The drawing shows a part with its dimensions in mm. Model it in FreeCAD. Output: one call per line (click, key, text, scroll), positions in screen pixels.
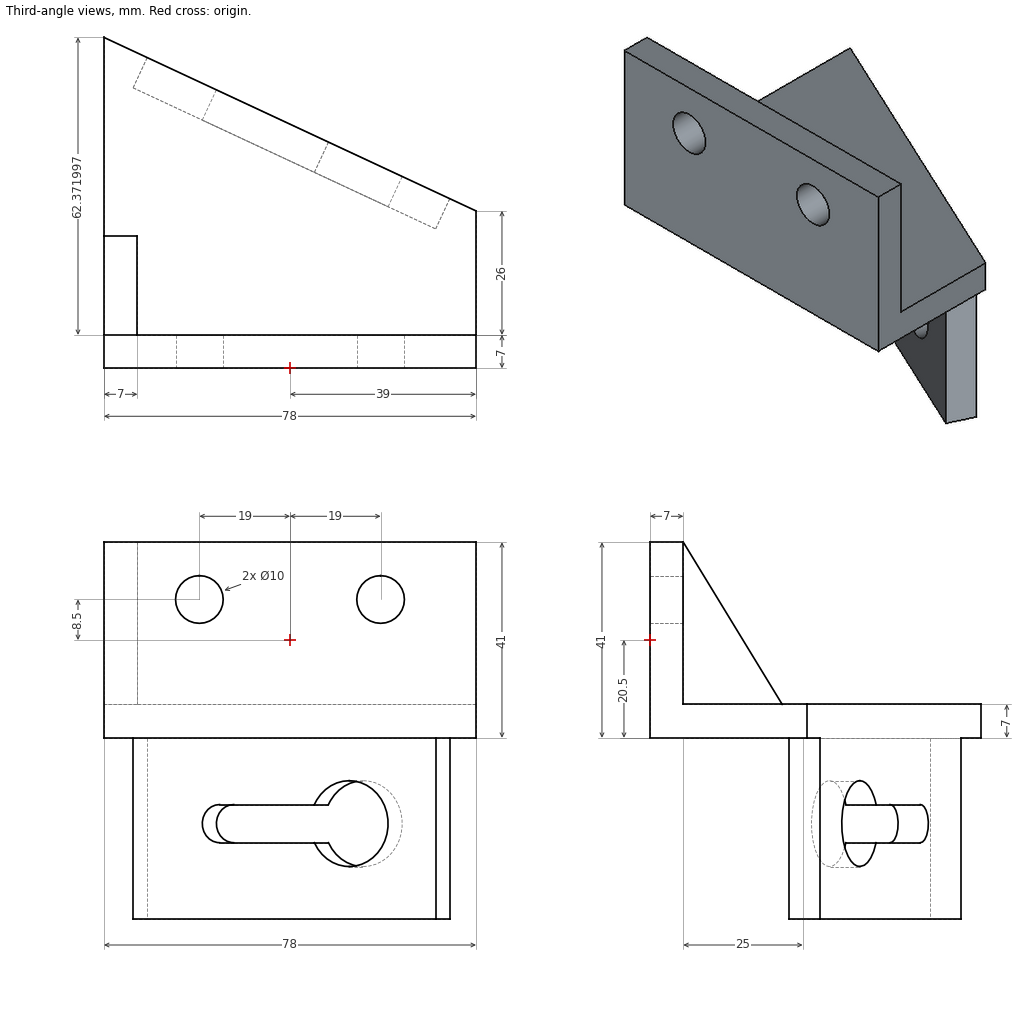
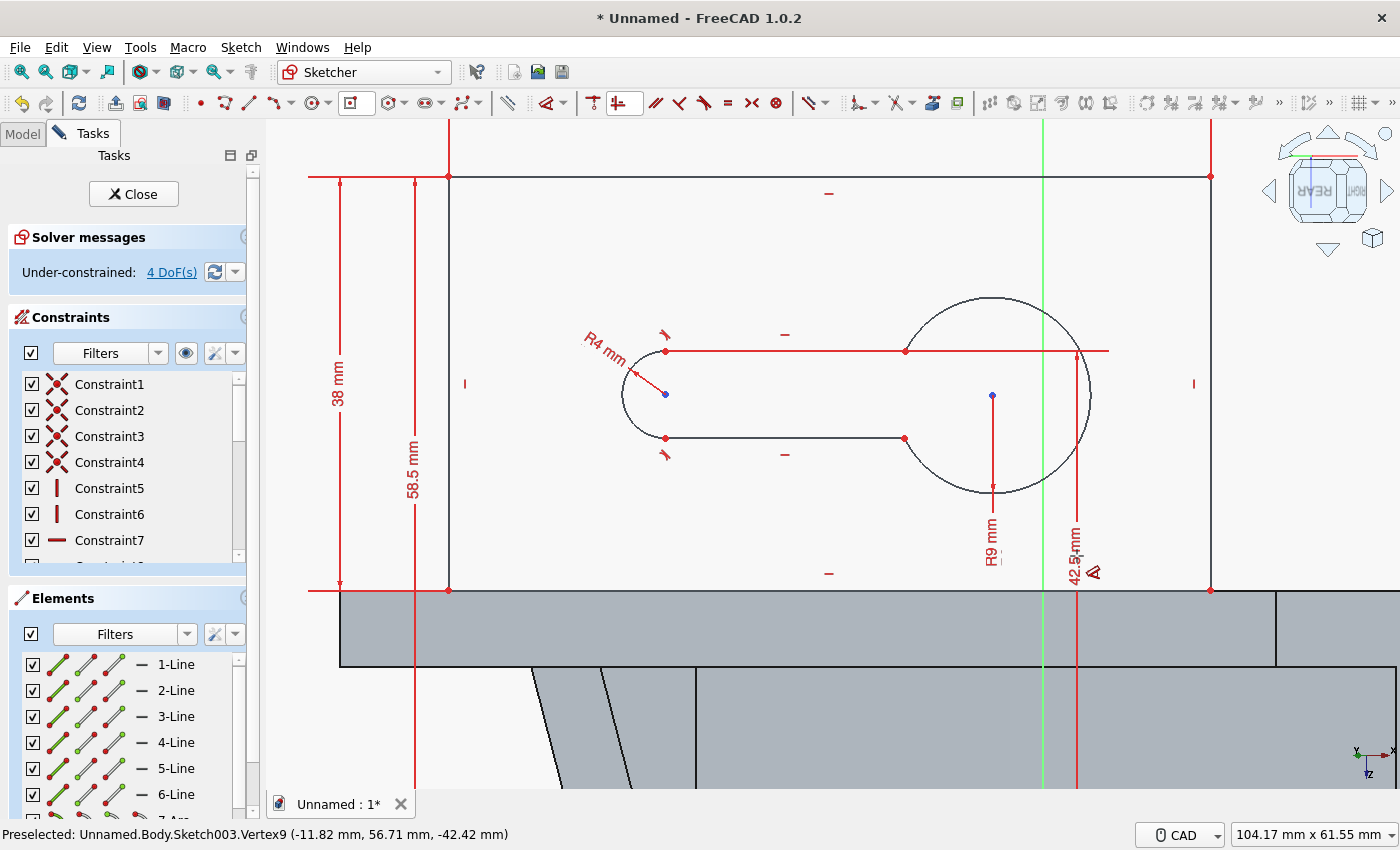
click(993, 396)
click(1077, 494)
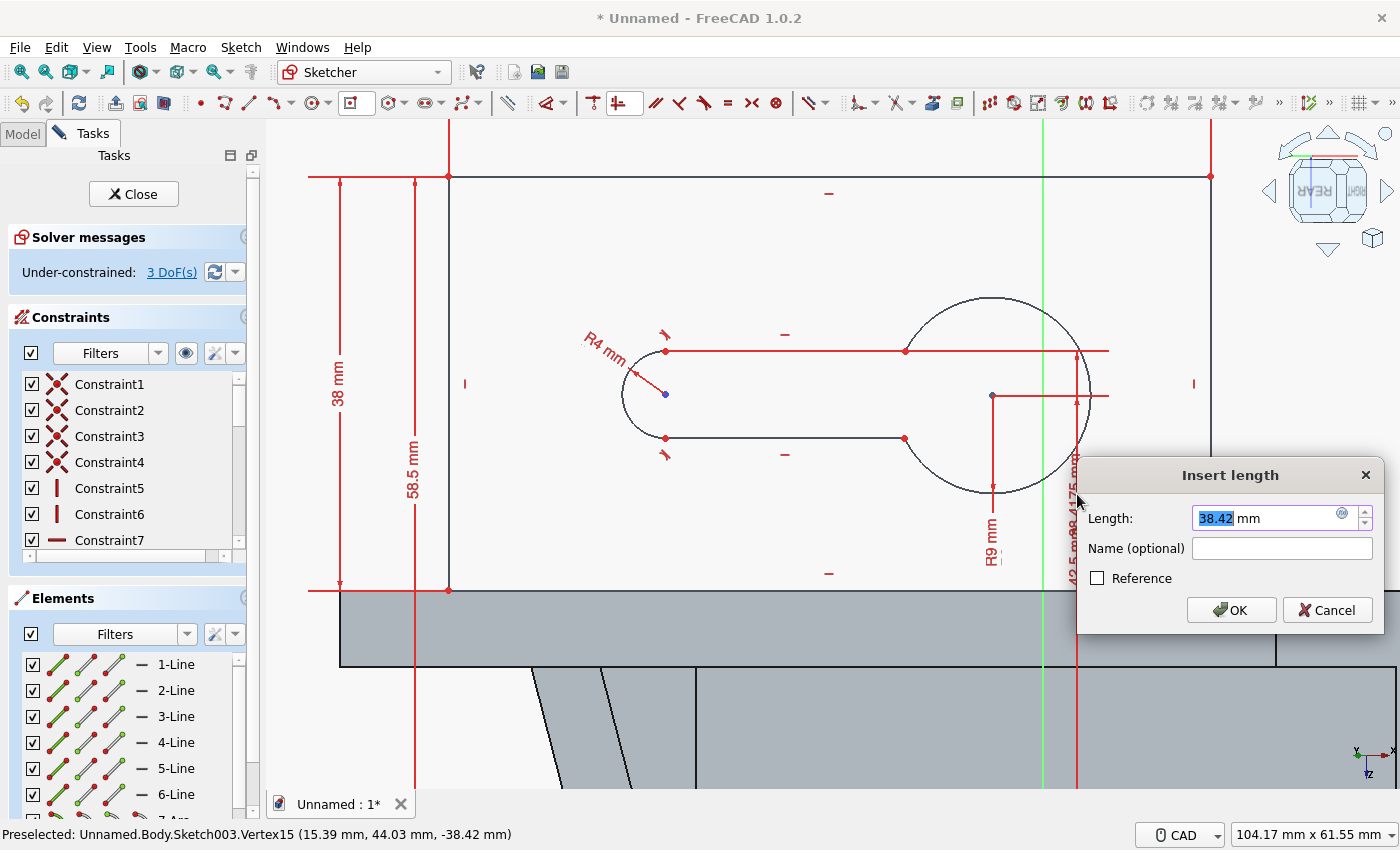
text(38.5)
key(Return)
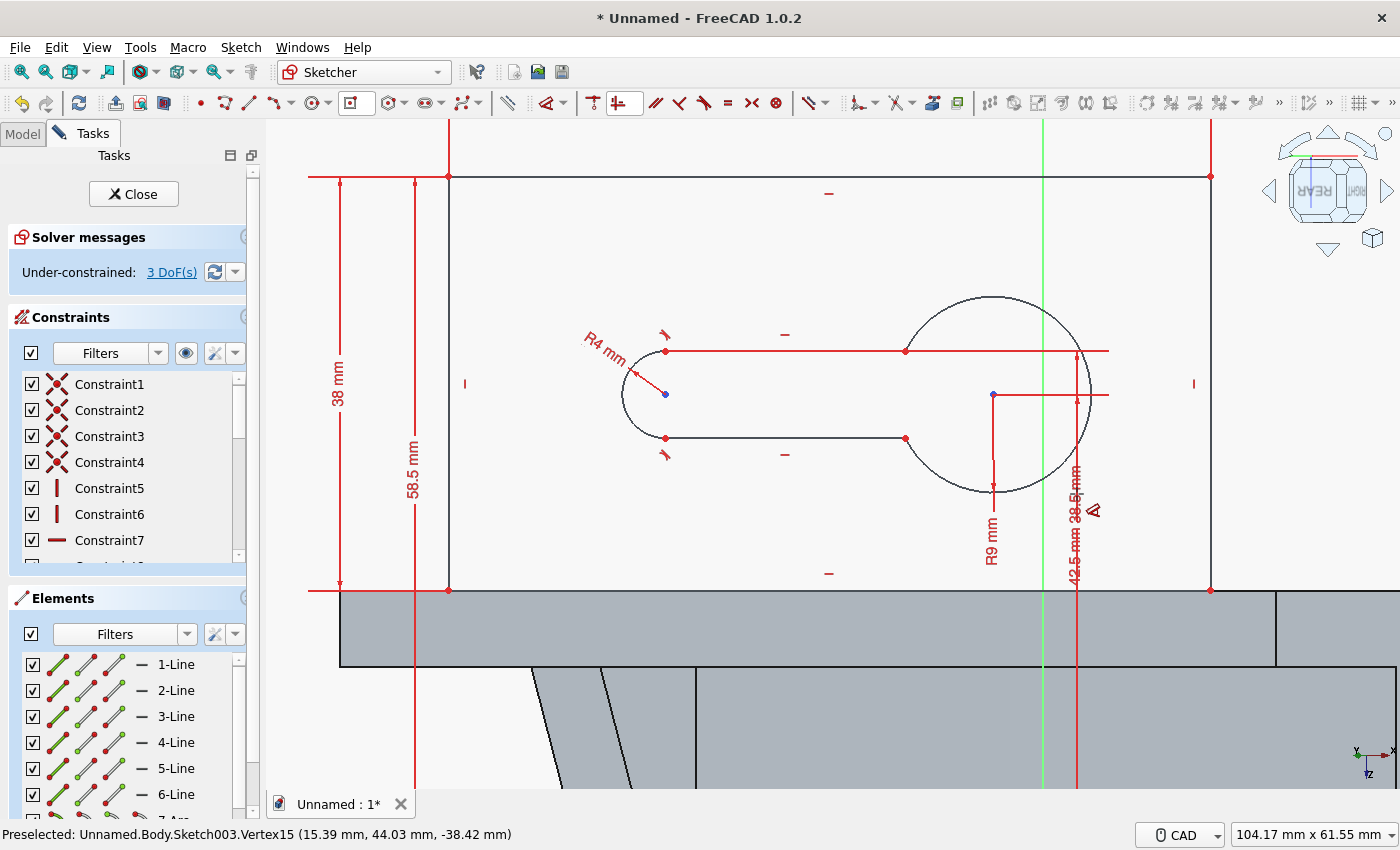
click(738, 351)
click(786, 317)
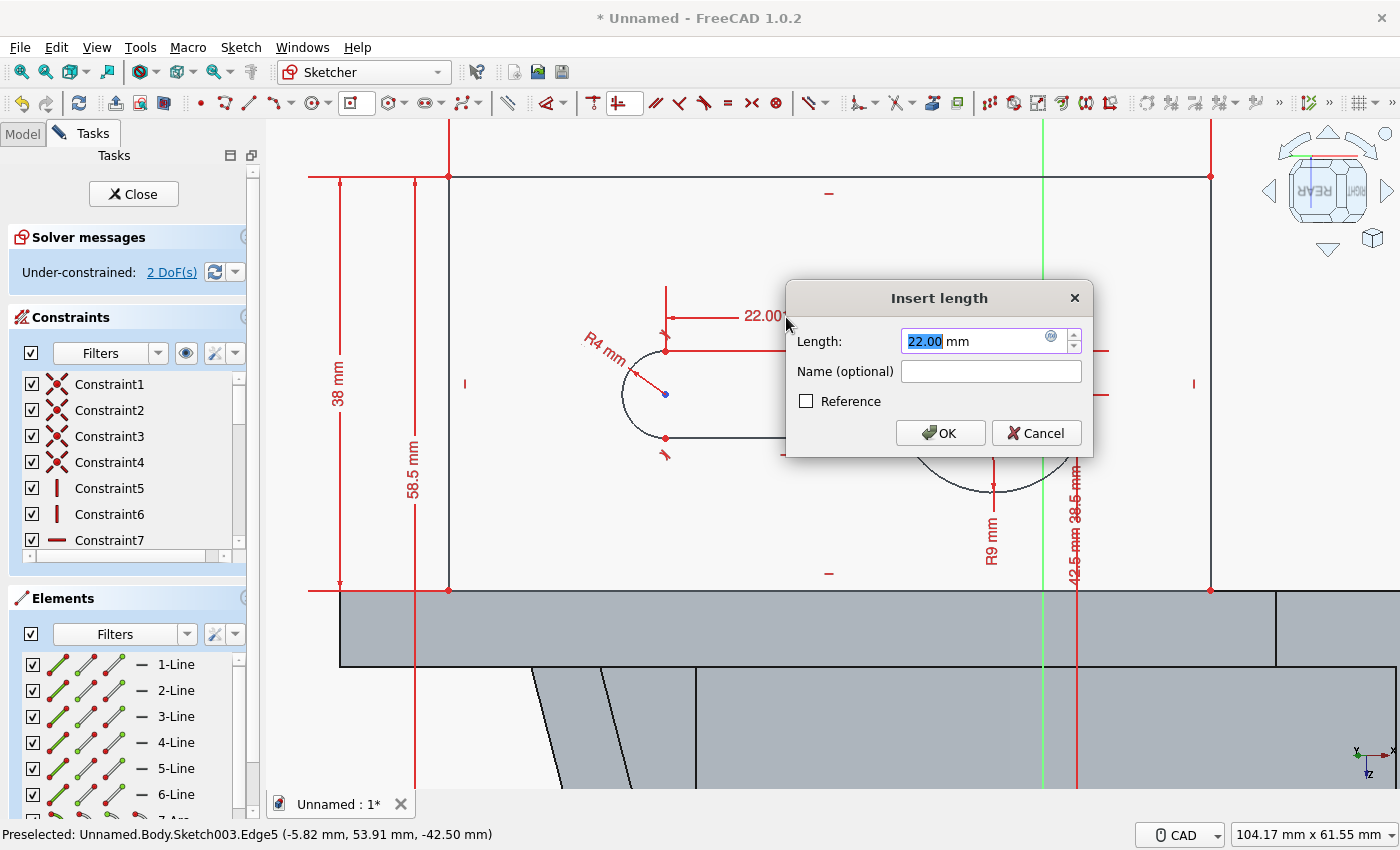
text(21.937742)
key(Return)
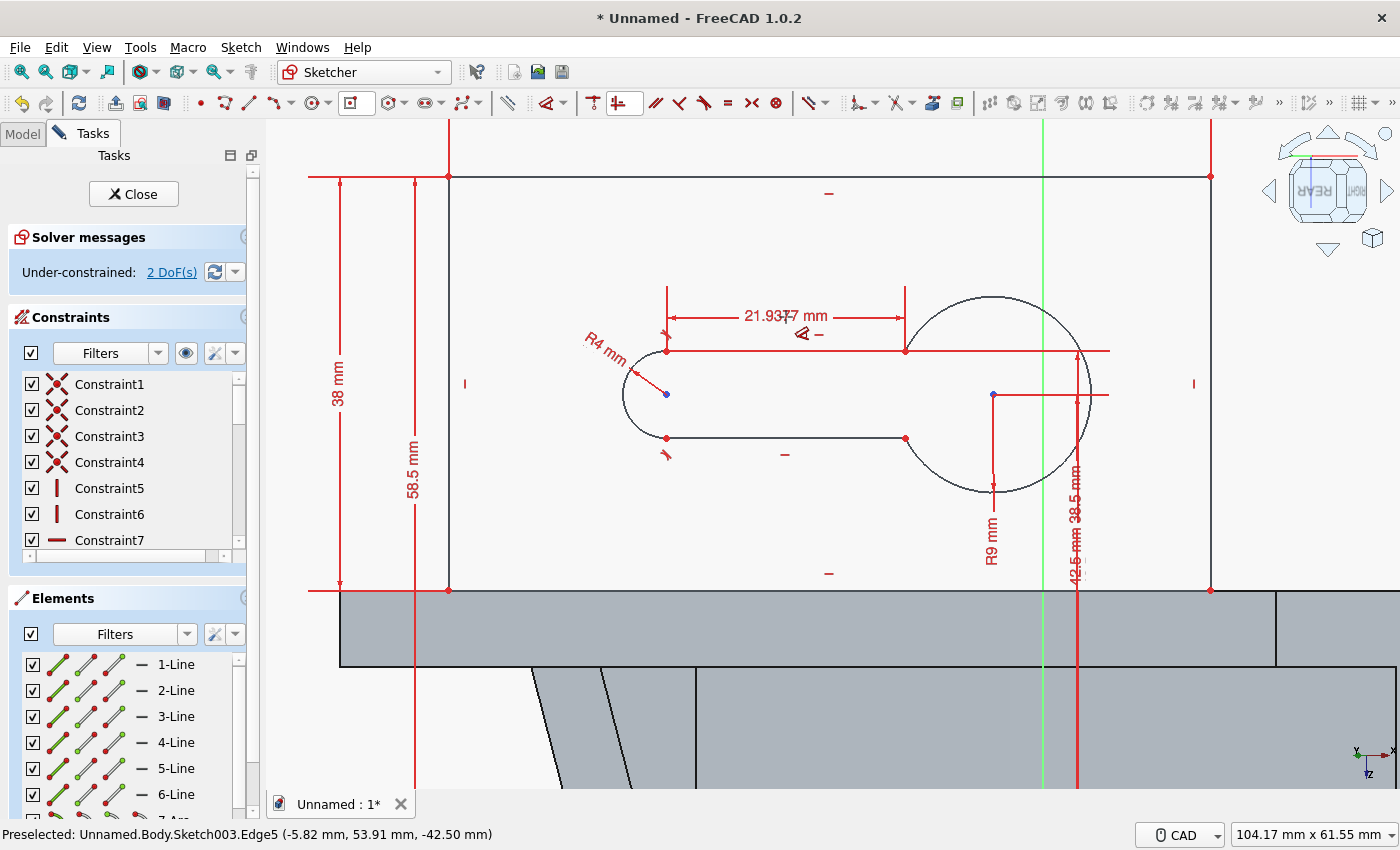
click(993, 395)
click(1018, 361)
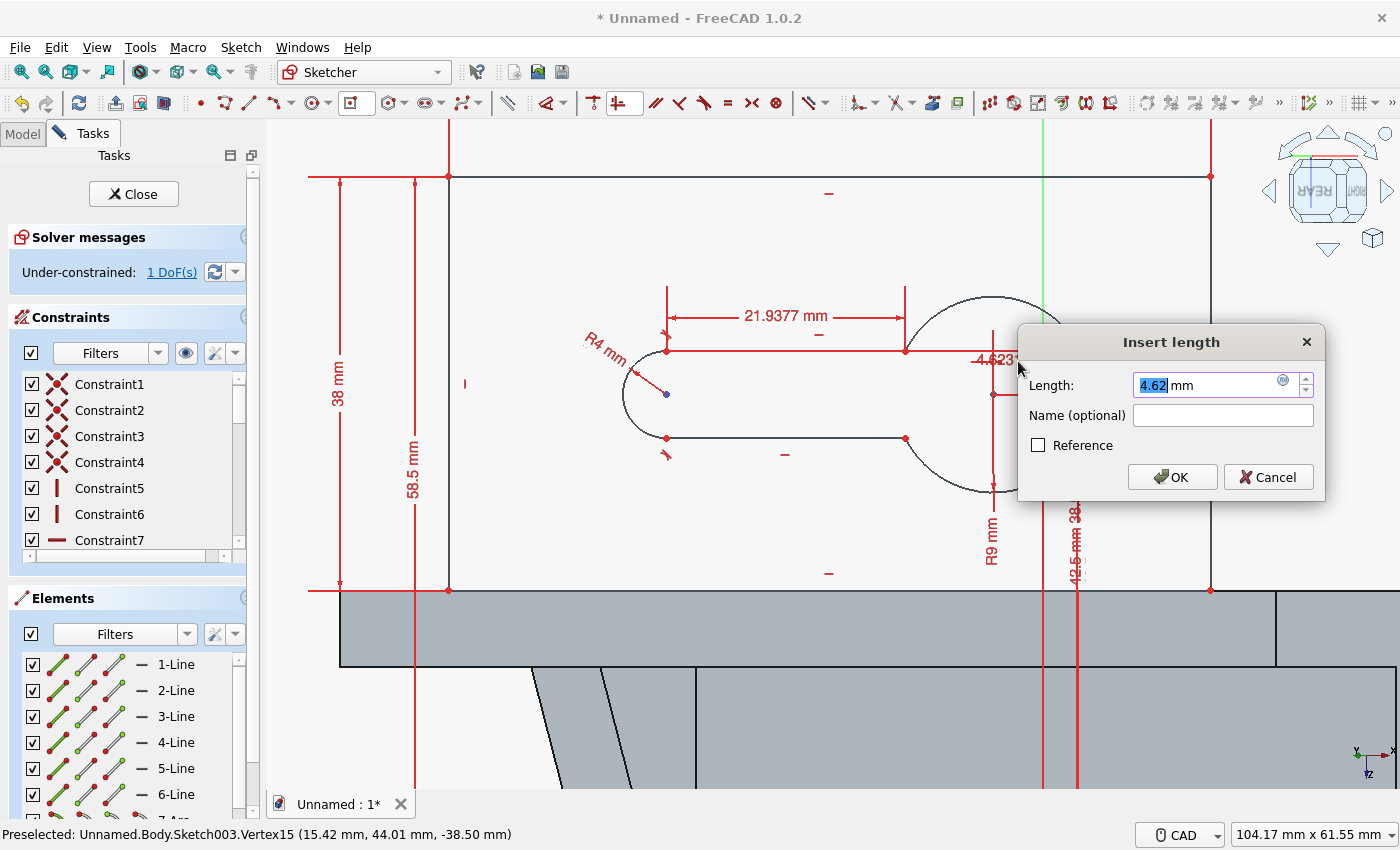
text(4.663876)
key(Return)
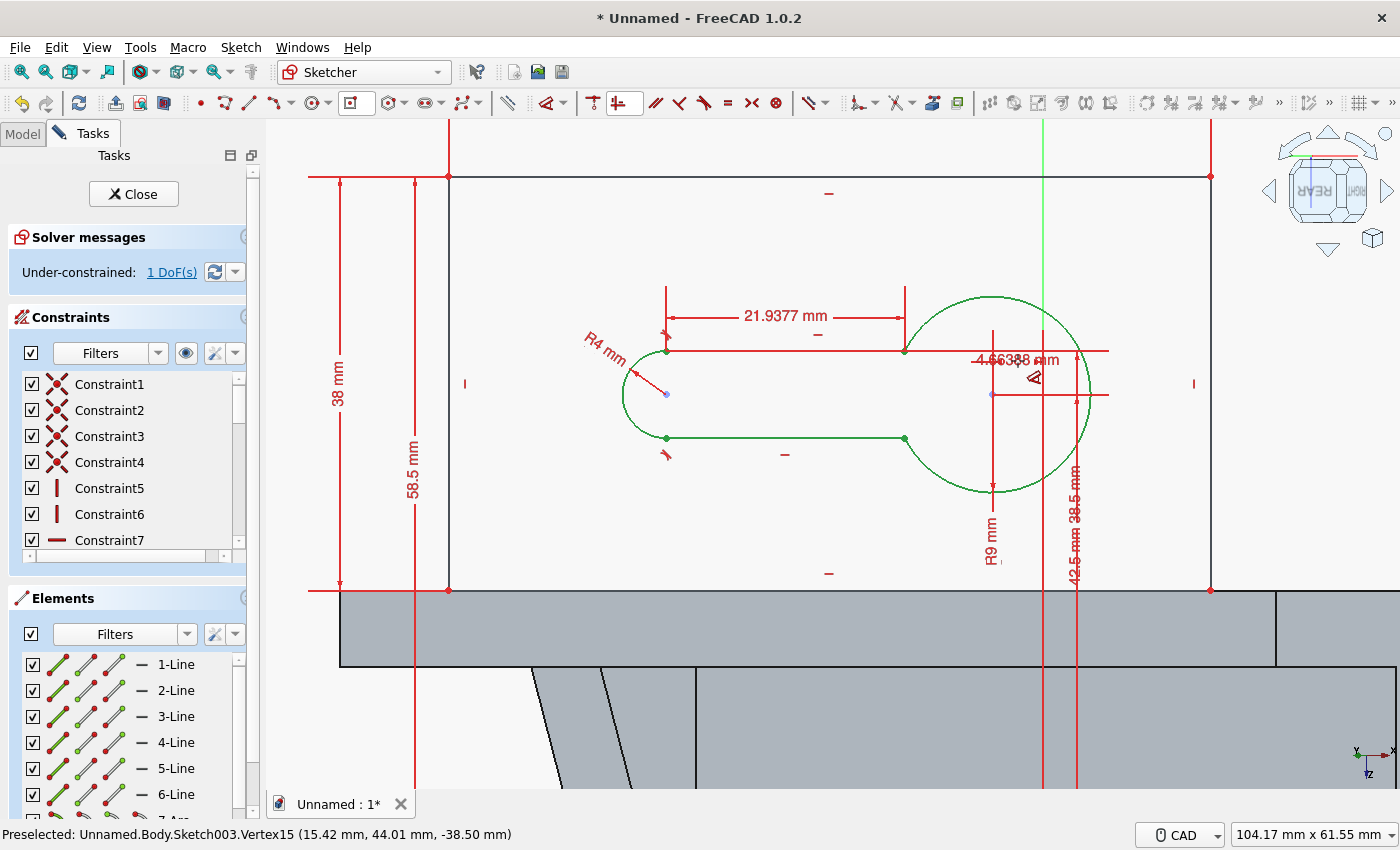
click(449, 177)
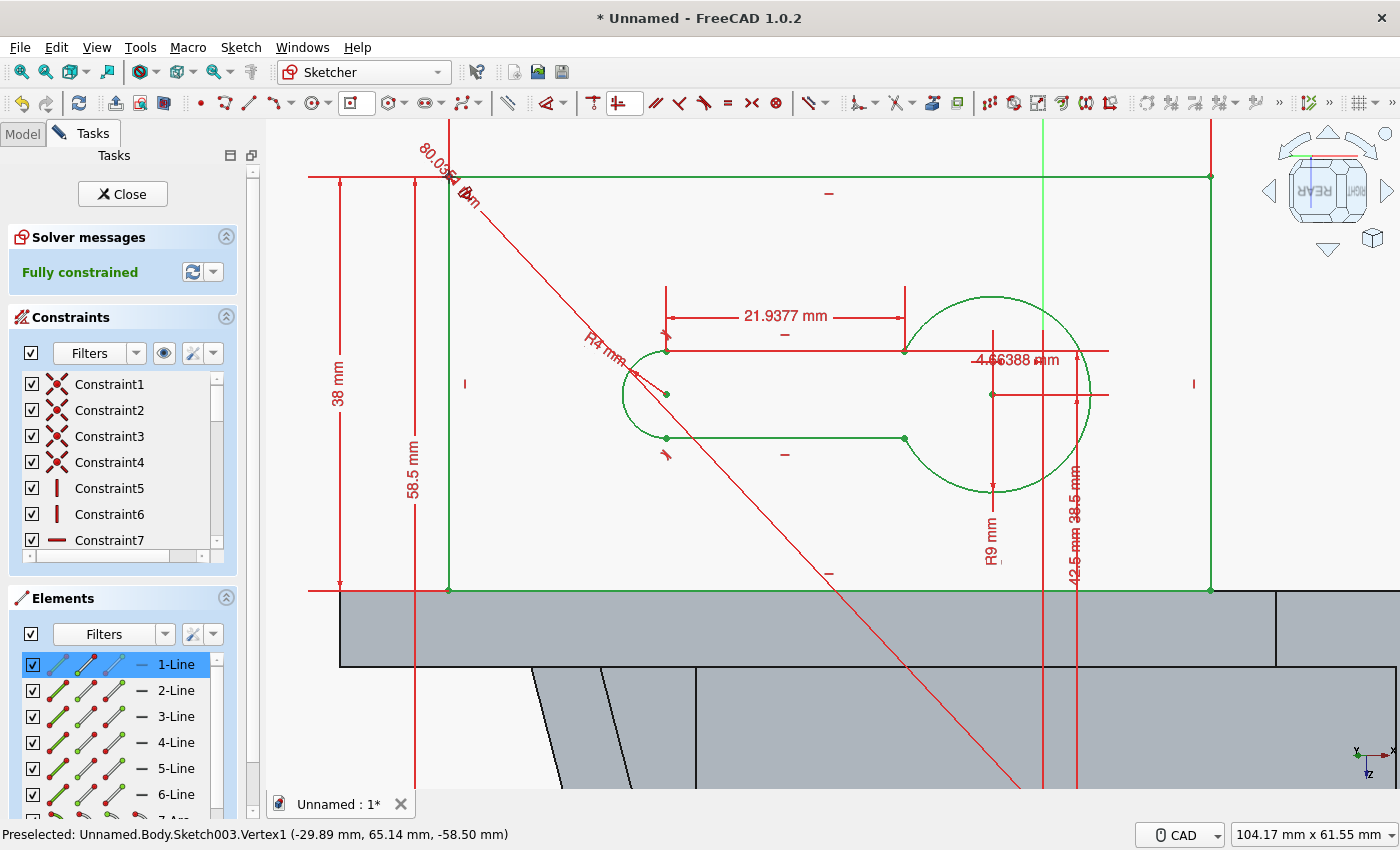
key(Escape)
key(Escape)